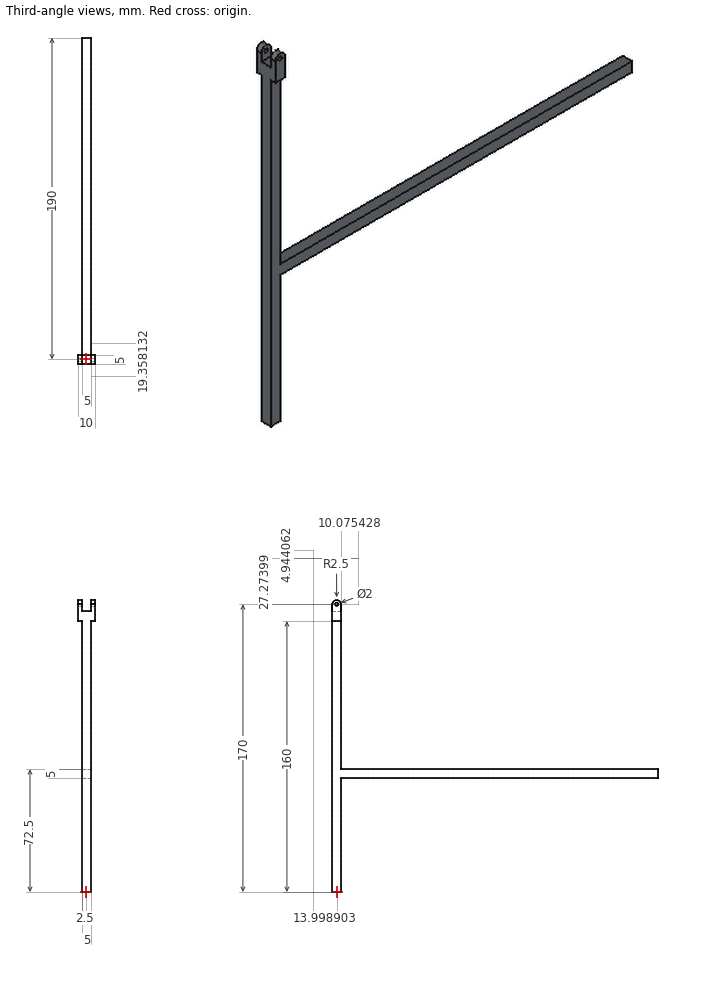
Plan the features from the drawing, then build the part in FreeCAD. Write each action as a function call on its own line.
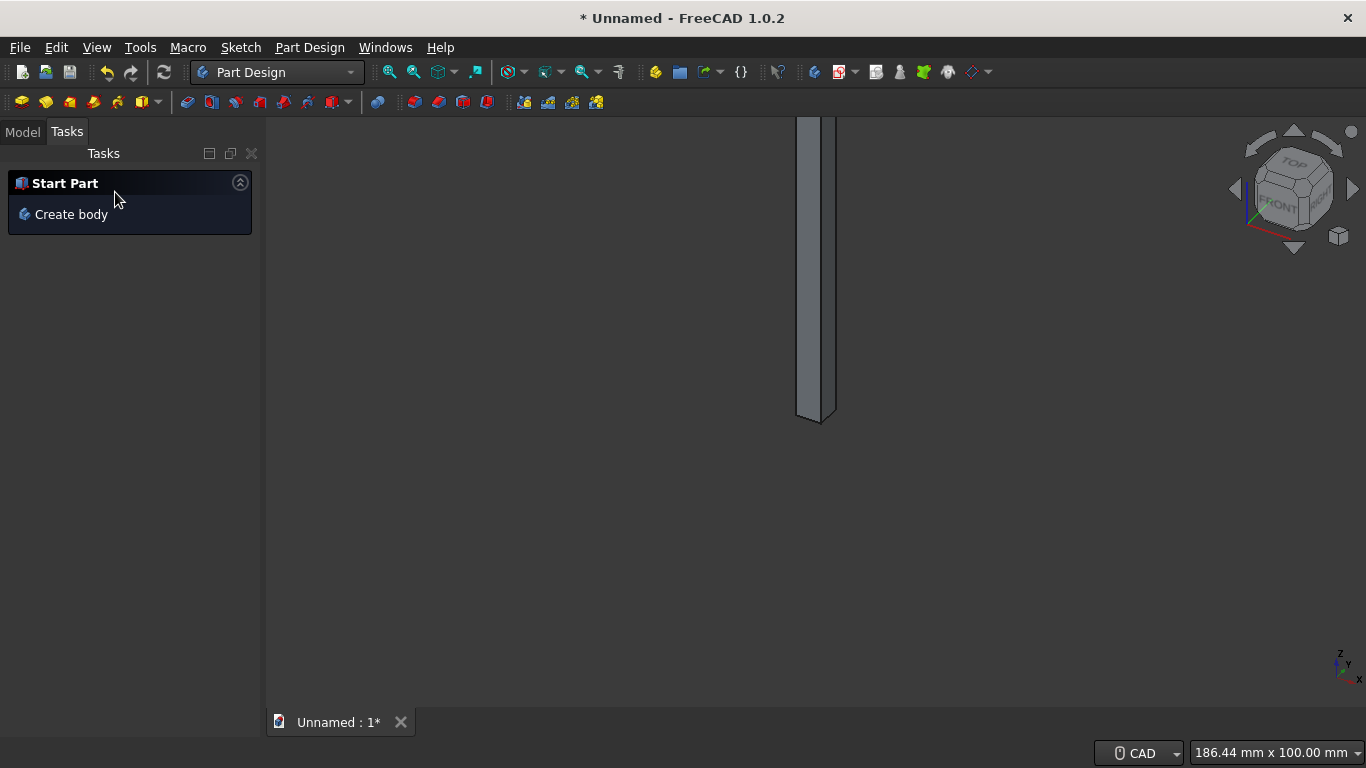
click(390, 72)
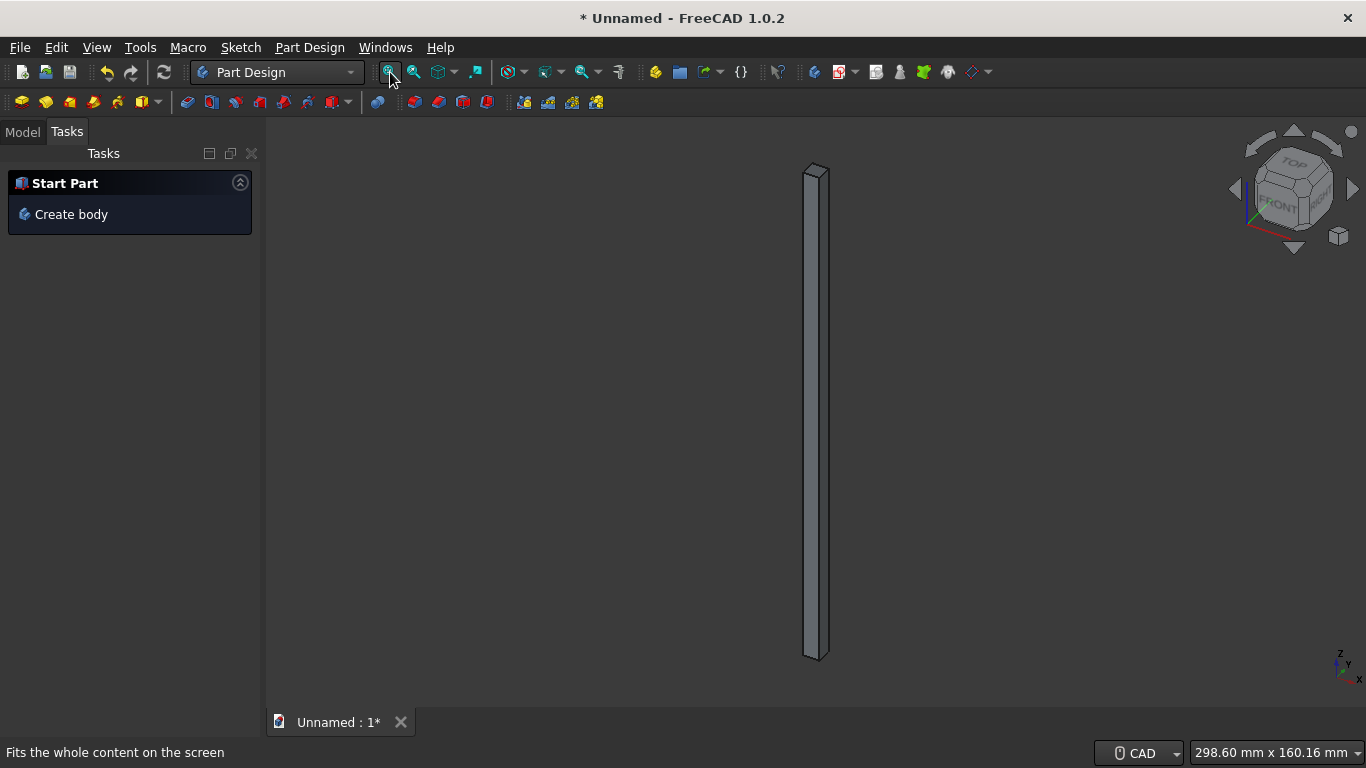
key(0)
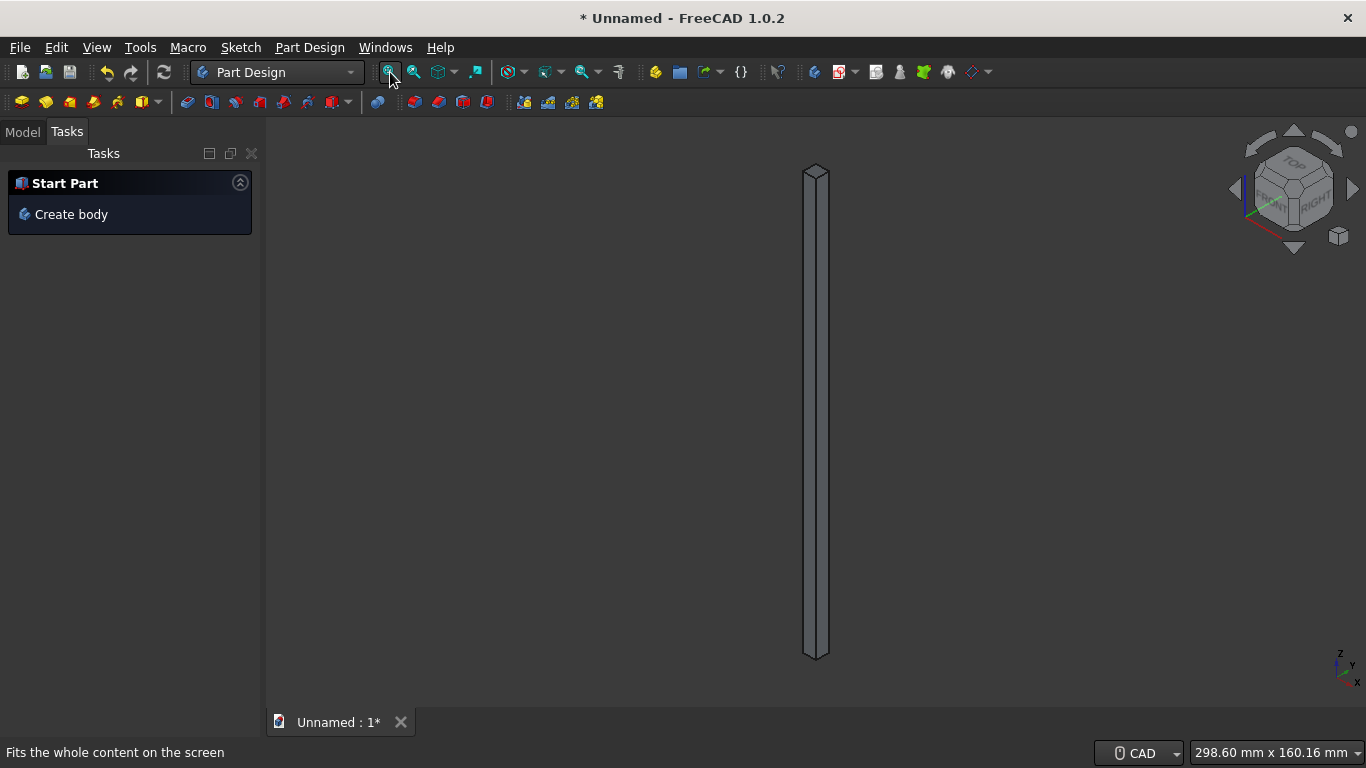
key(2)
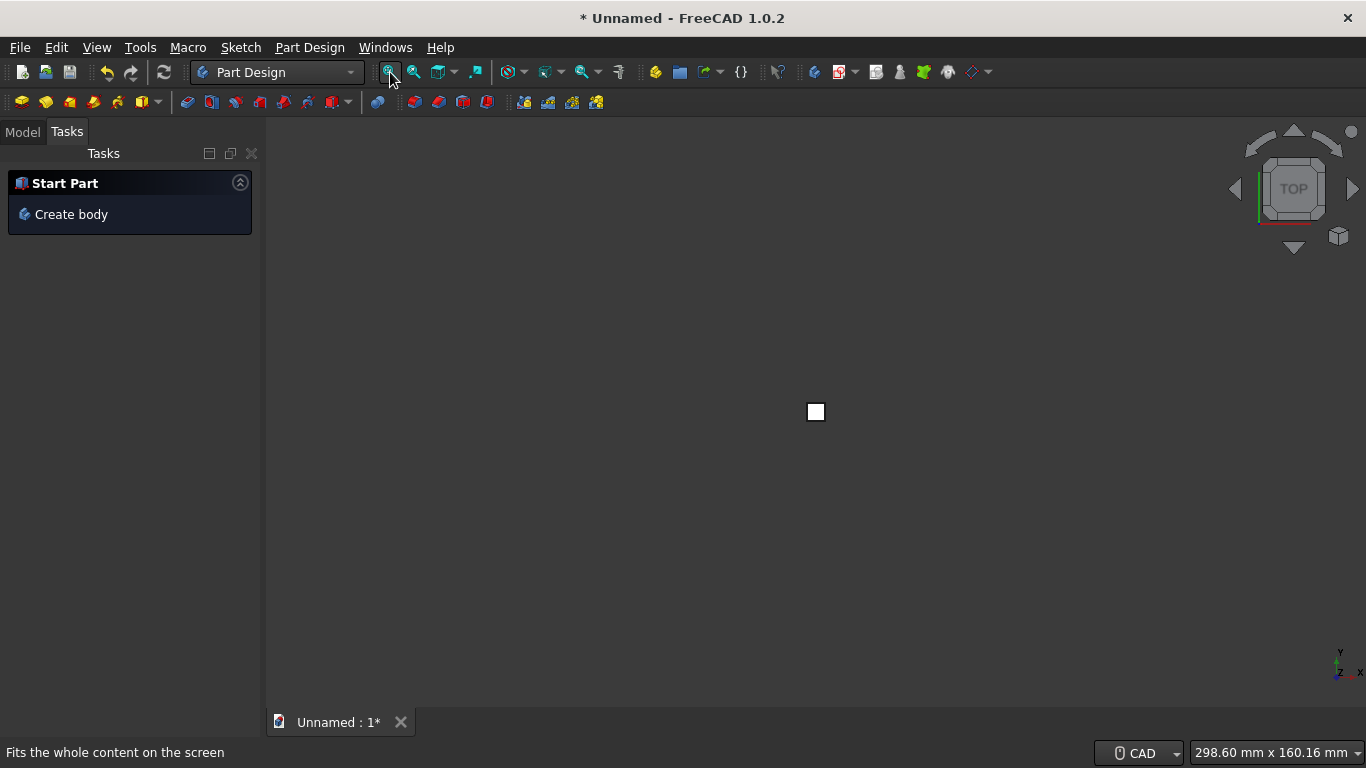
click(390, 72)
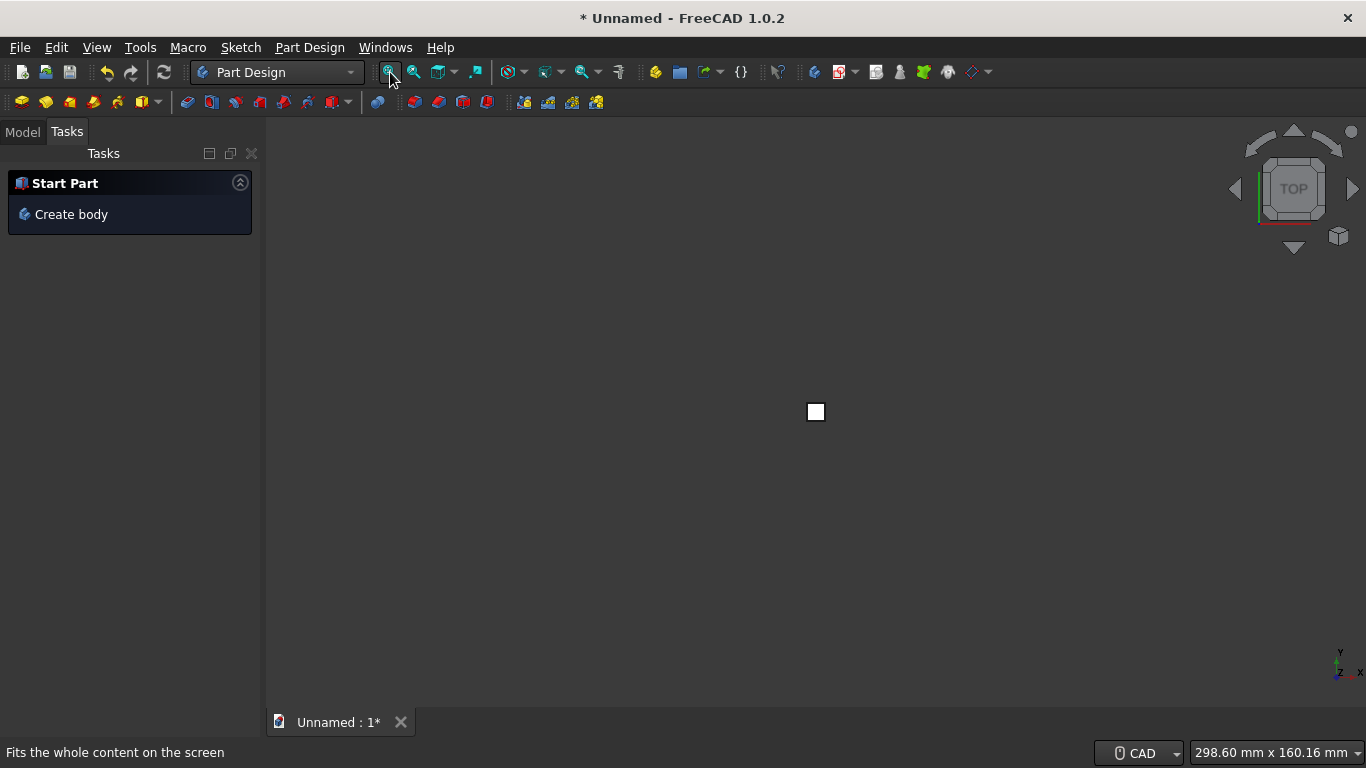
click(816, 411)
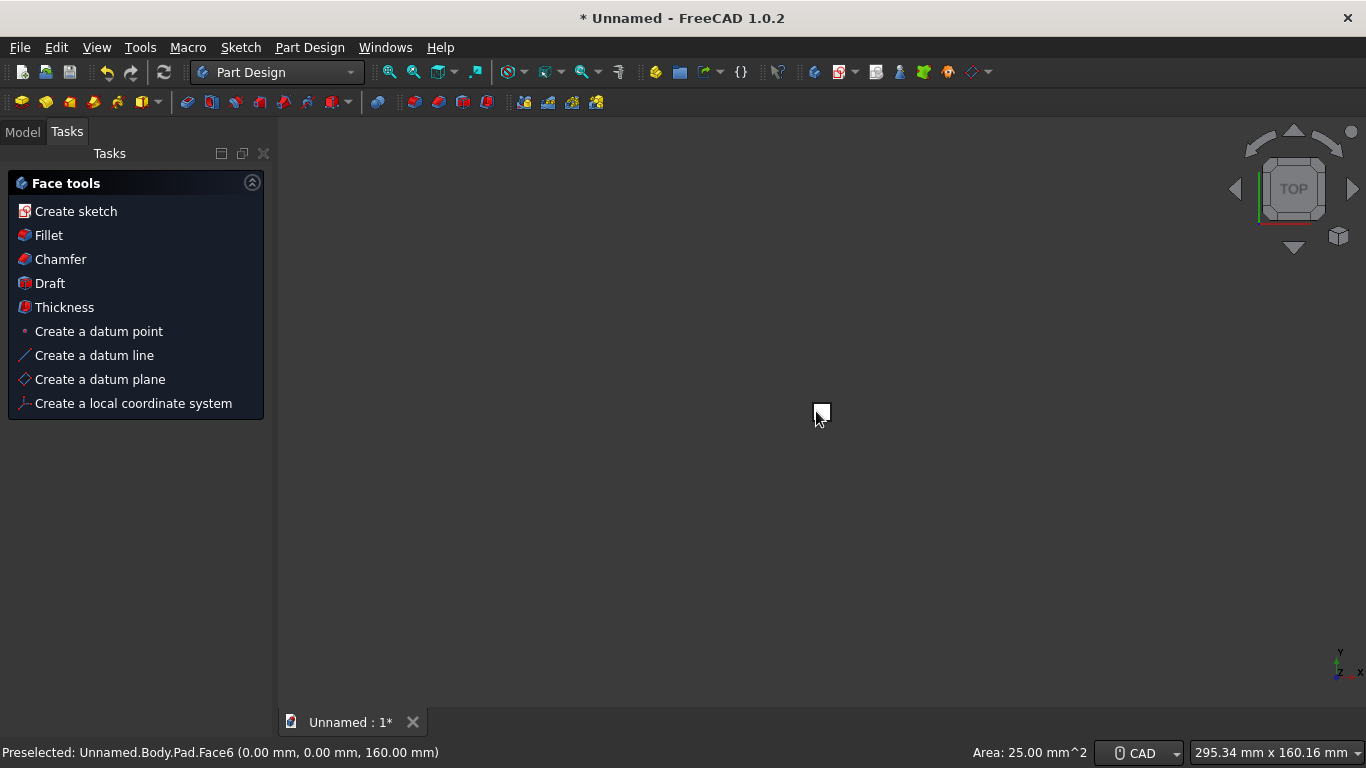
click(840, 72)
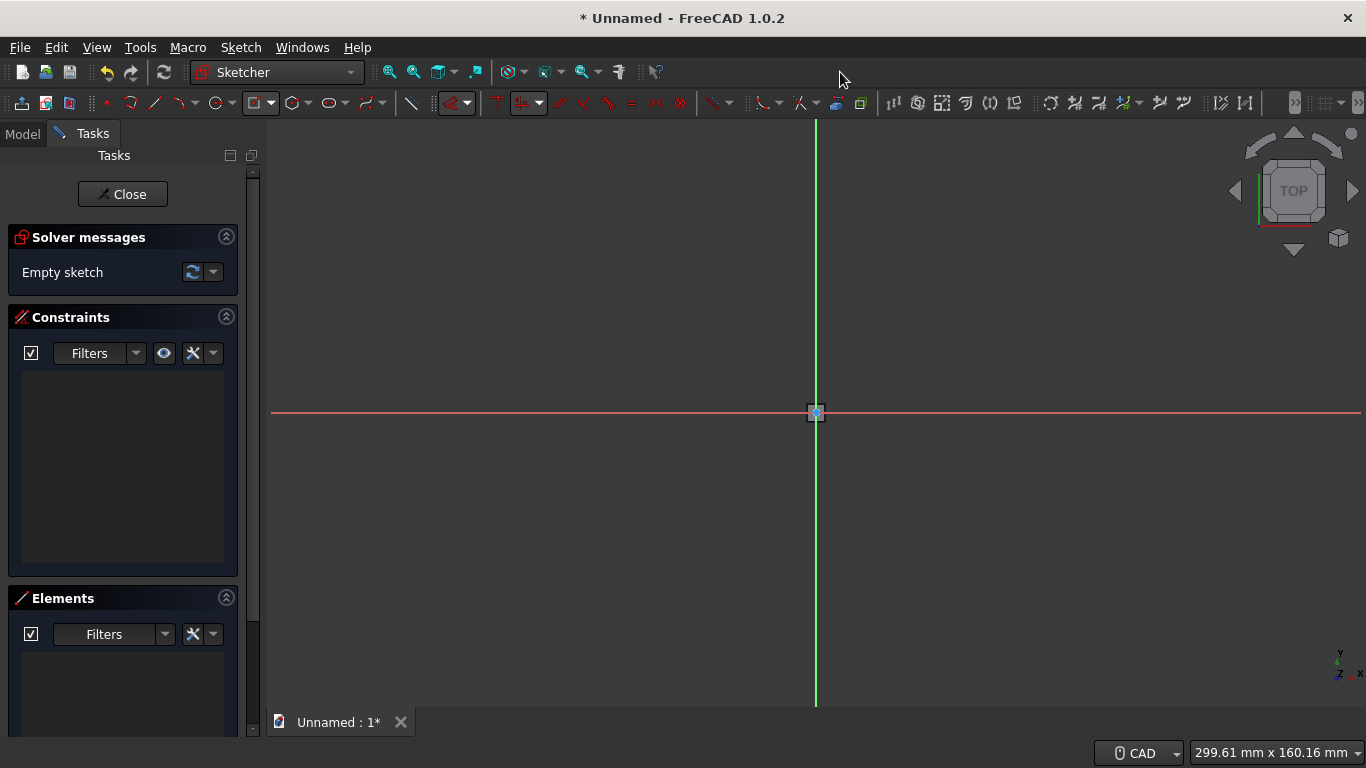
scroll(820, 413, up, 14)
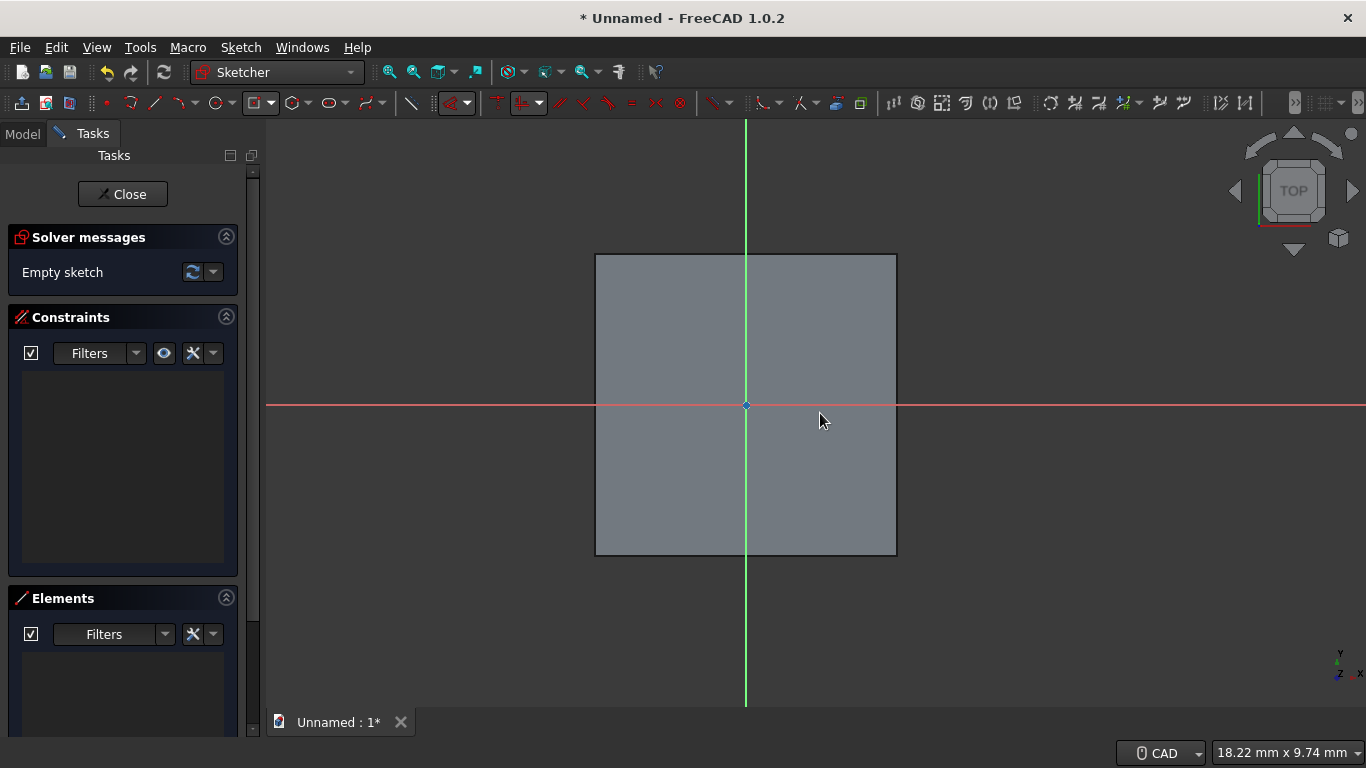
click(254, 104)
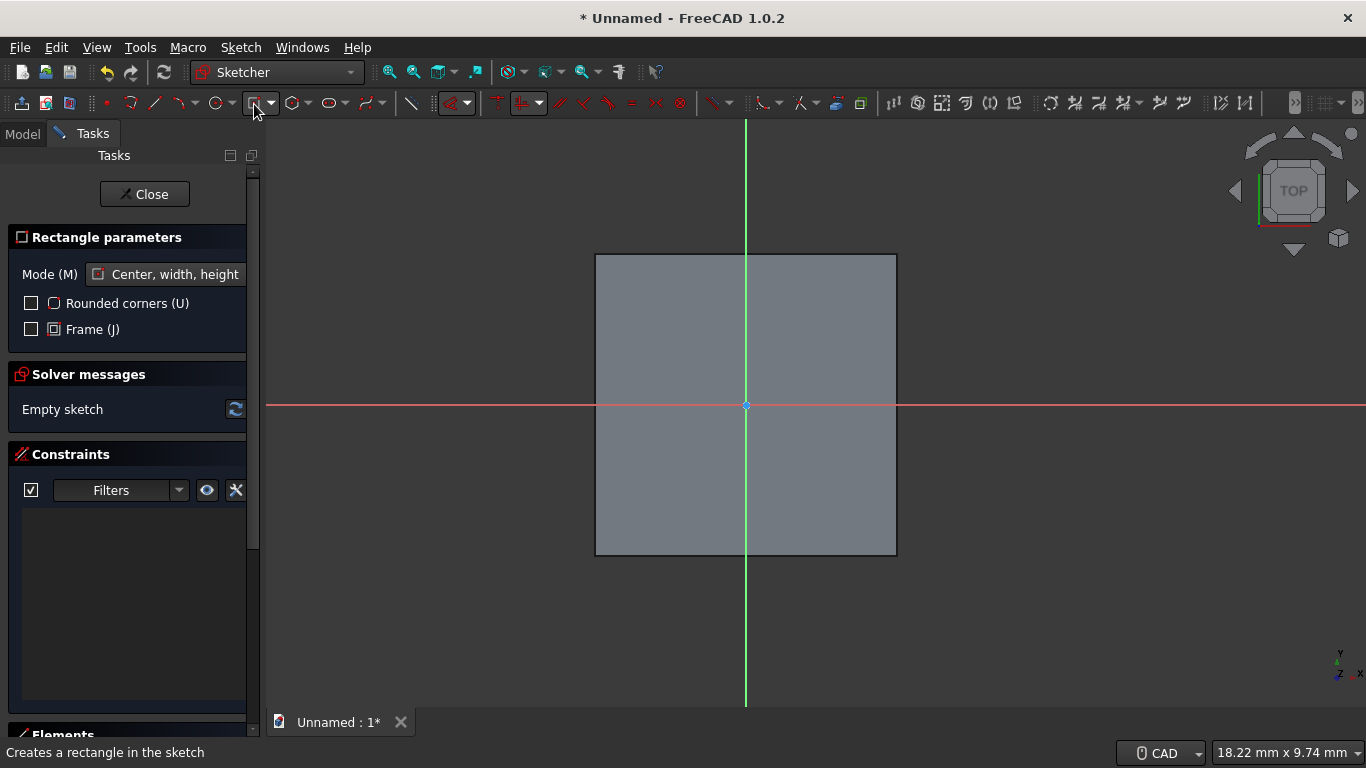
click(746, 405)
click(1048, 254)
key(Escape)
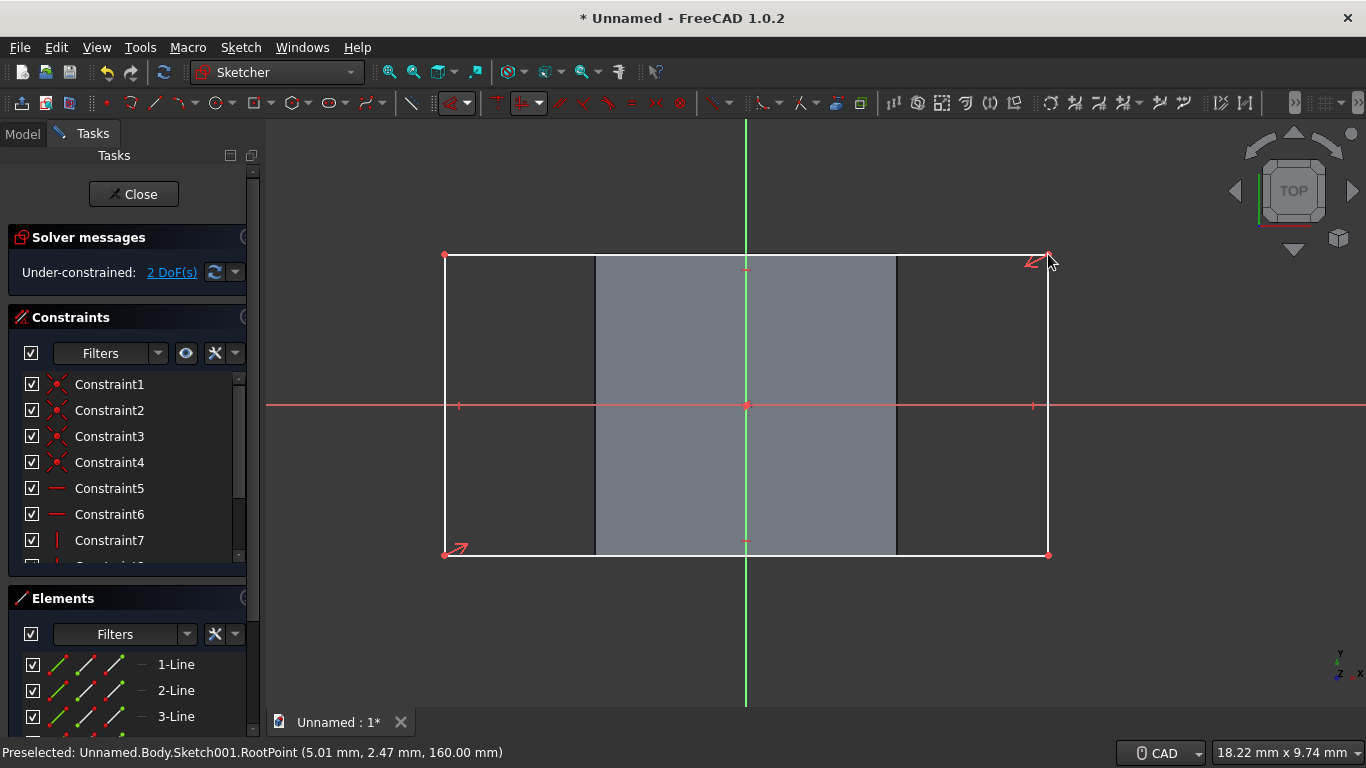
click(1048, 465)